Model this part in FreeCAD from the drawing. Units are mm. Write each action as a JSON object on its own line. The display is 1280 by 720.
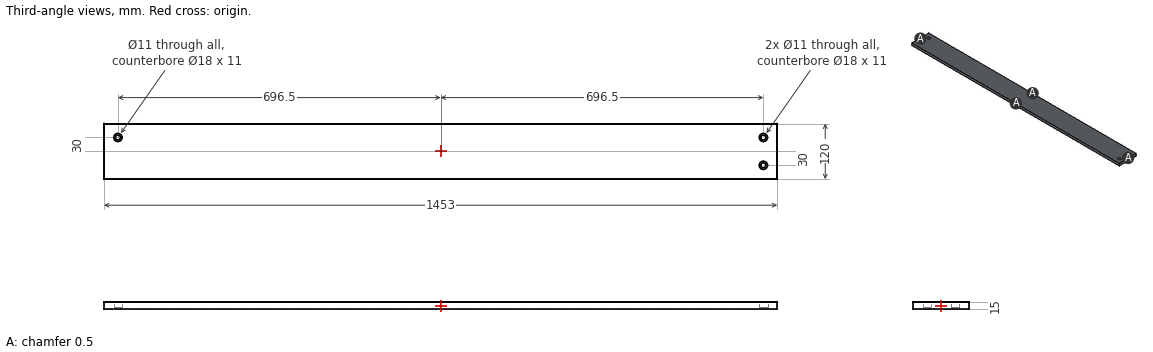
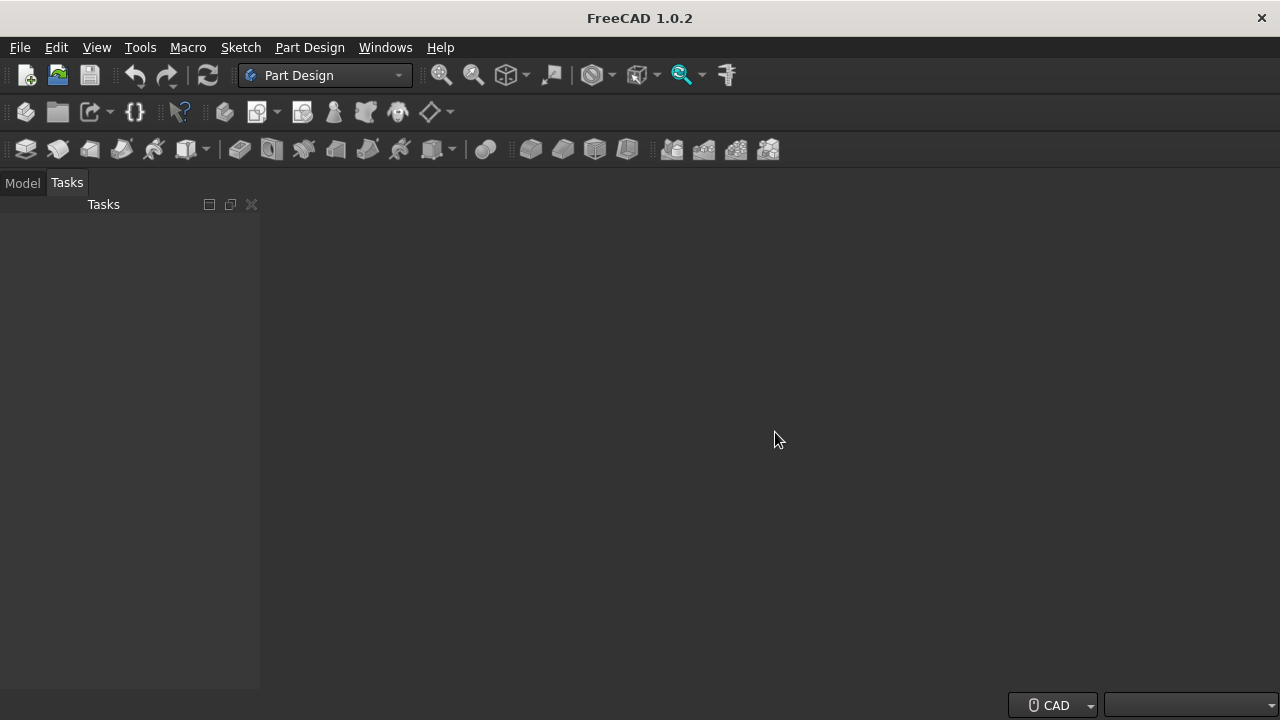
{"action": "left_click", "coordinate": [26, 76]}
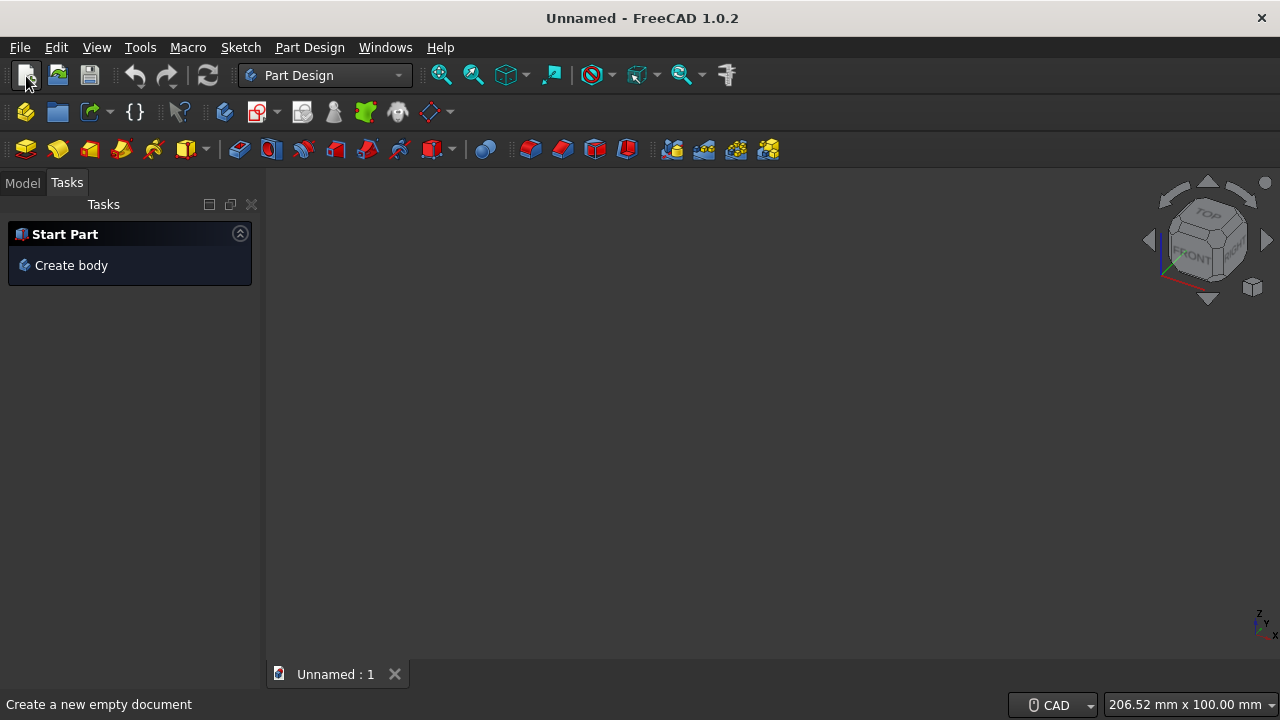
{"action": "left_click", "coordinate": [258, 112]}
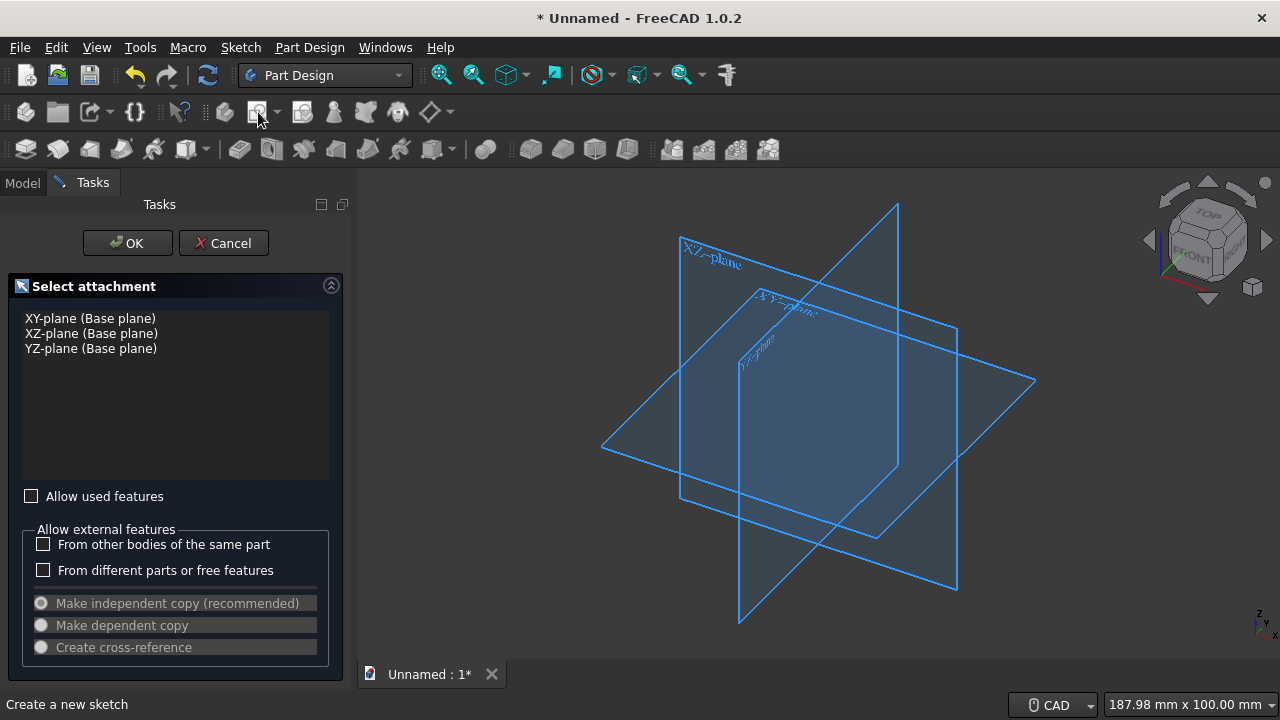
{"action": "left_click", "coordinate": [82, 318]}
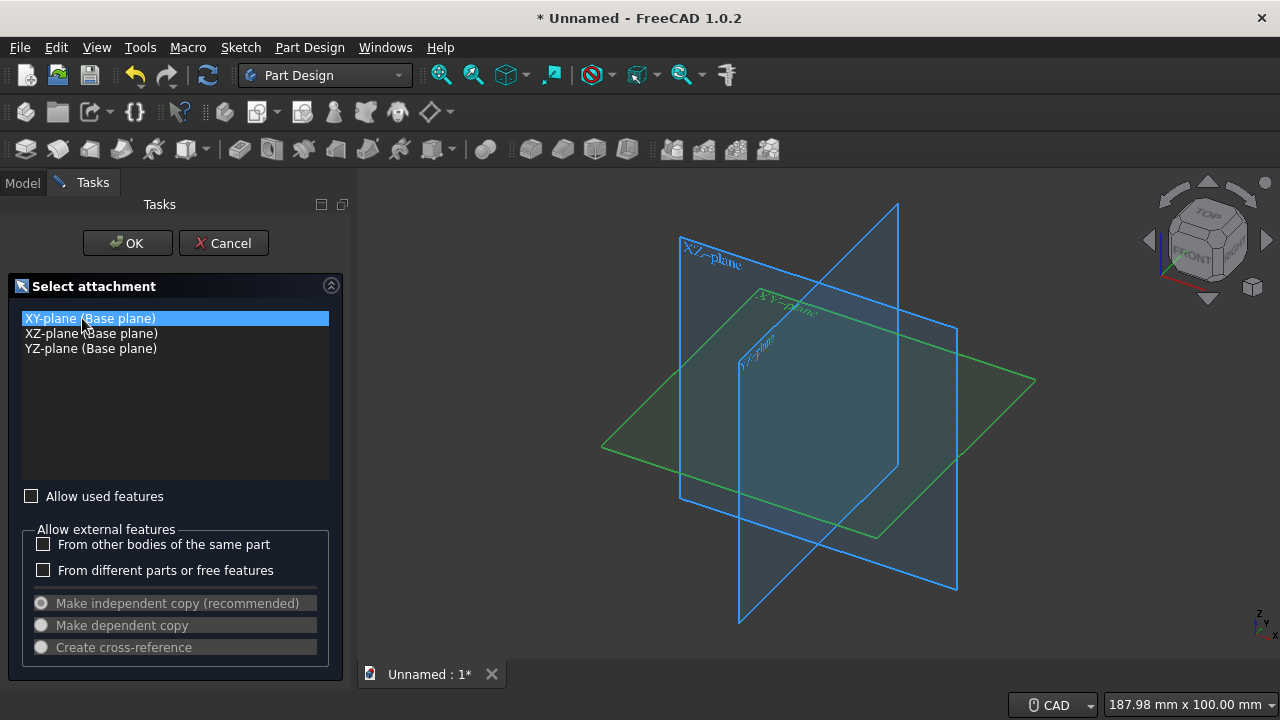
{"action": "left_click", "coordinate": [128, 243]}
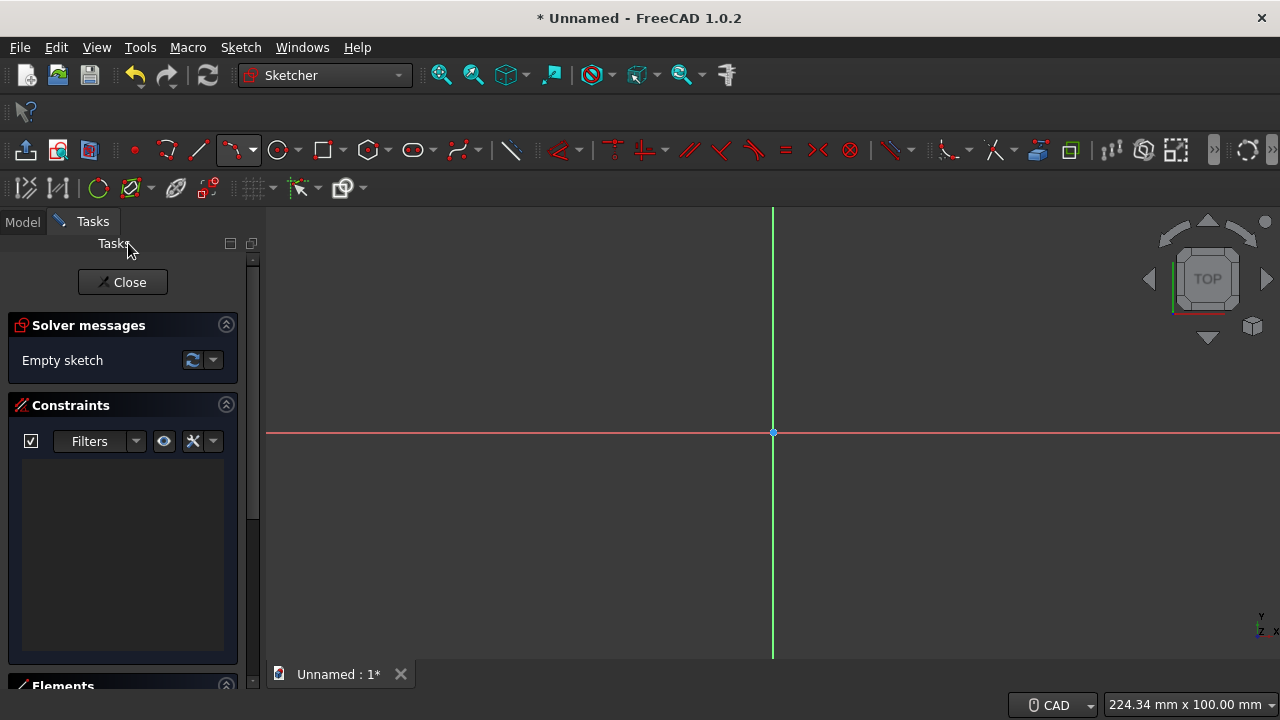
{"action": "scroll", "coordinate": [698, 433], "scroll_direction": "down", "scroll_amount": 12}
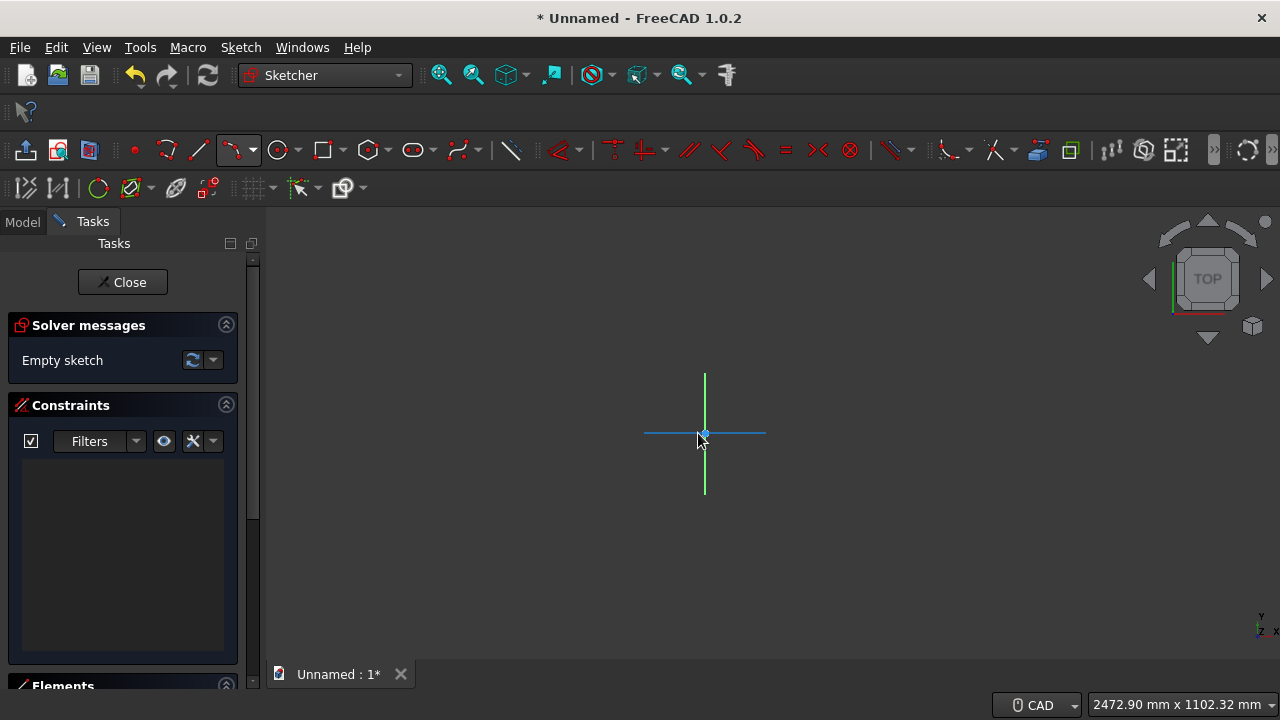
{"action": "left_click", "coordinate": [346, 150]}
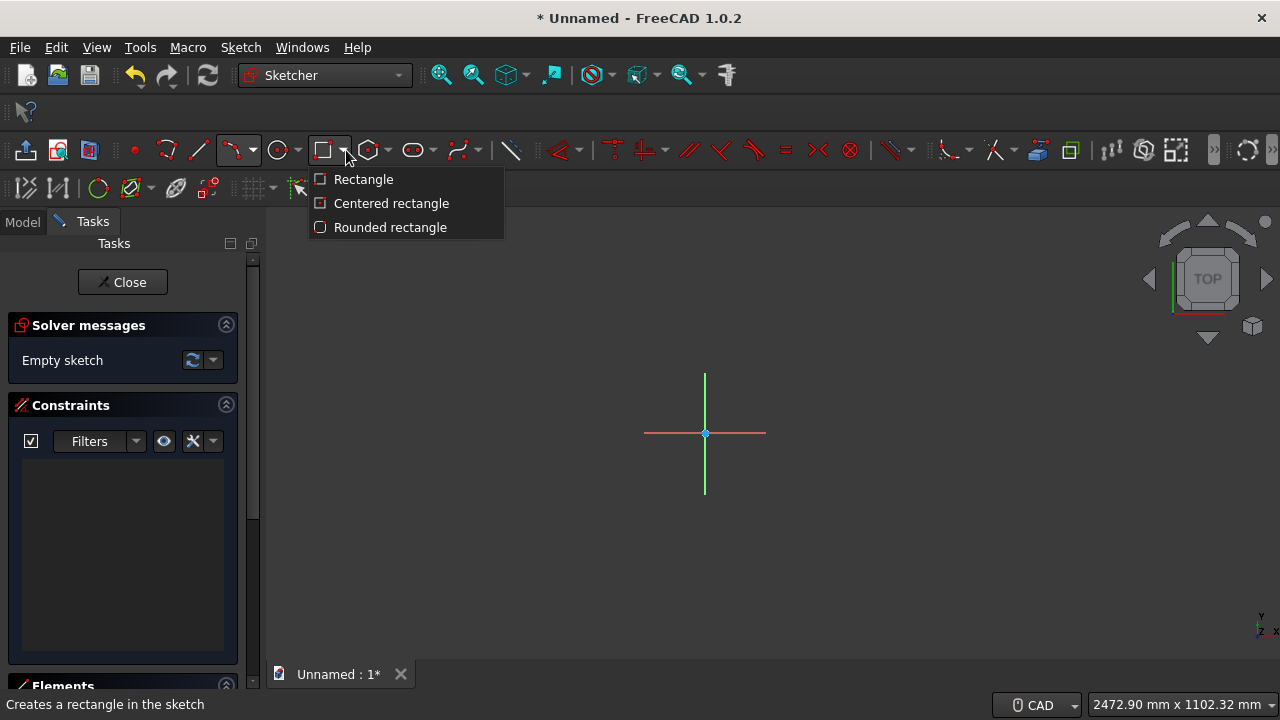
{"action": "left_click", "coordinate": [406, 203]}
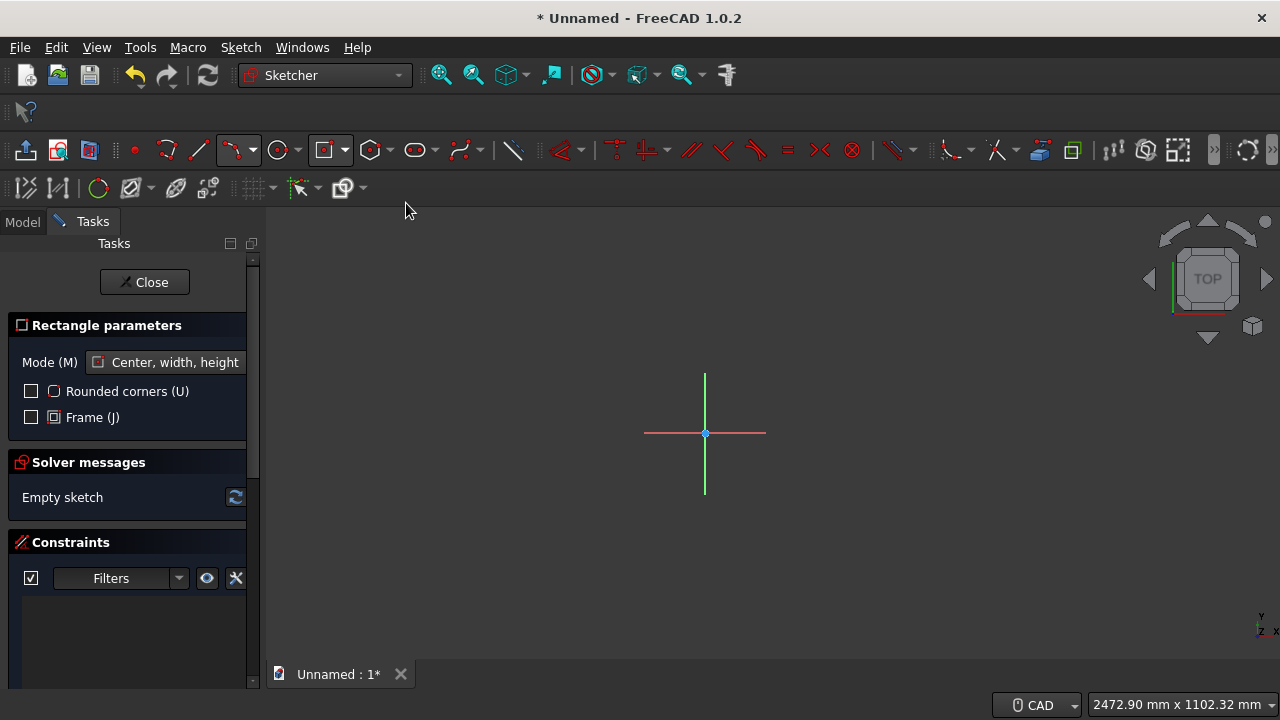
{"action": "left_click", "coordinate": [705, 433]}
{"action": "mouse_move", "coordinate": [1003, 409]}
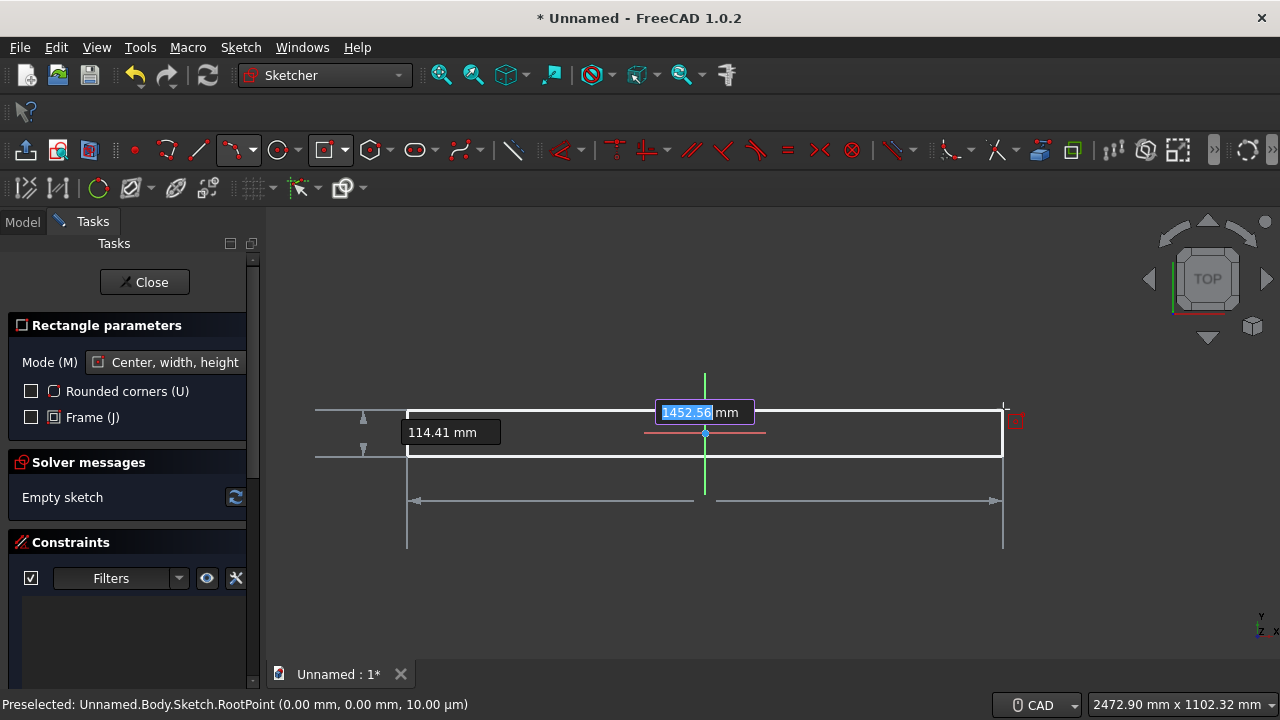
{"action": "type", "text": "1453"}
{"action": "key", "text": "Tab"}
{"action": "type", "text": "120"}
{"action": "key", "text": "Return"}
{"action": "key", "text": "Escape"}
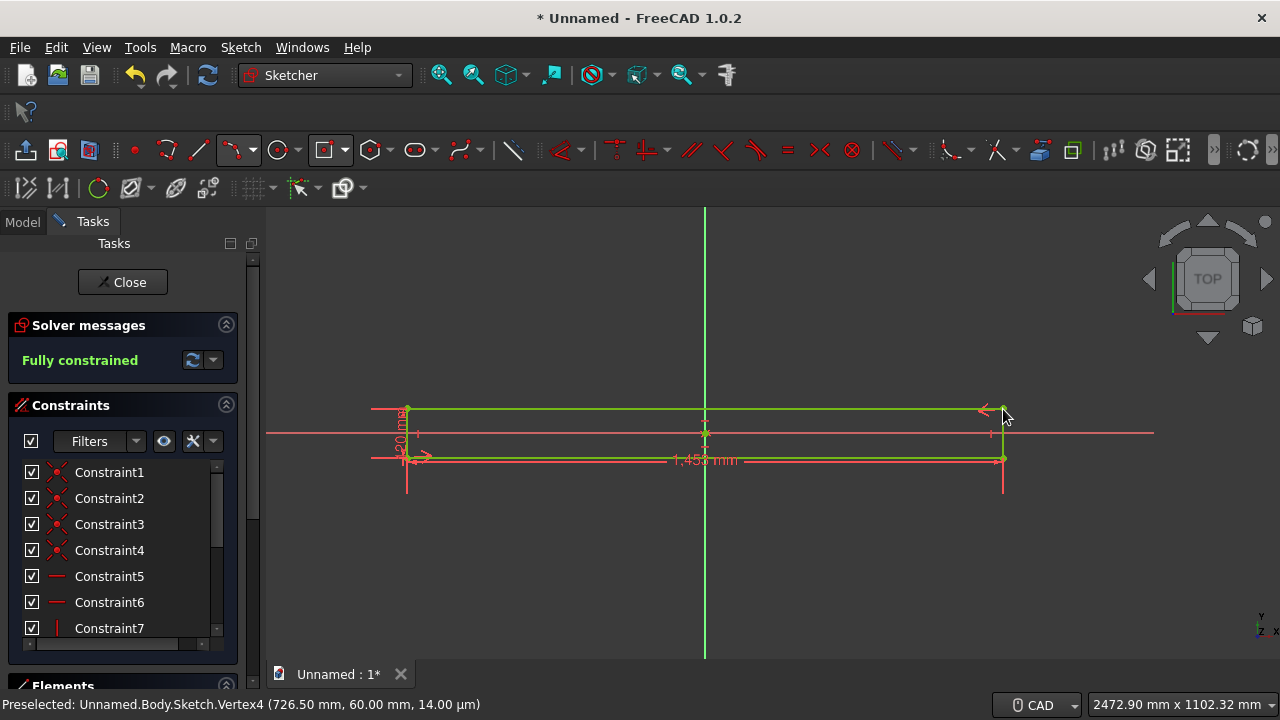
{"action": "left_click", "coordinate": [123, 282]}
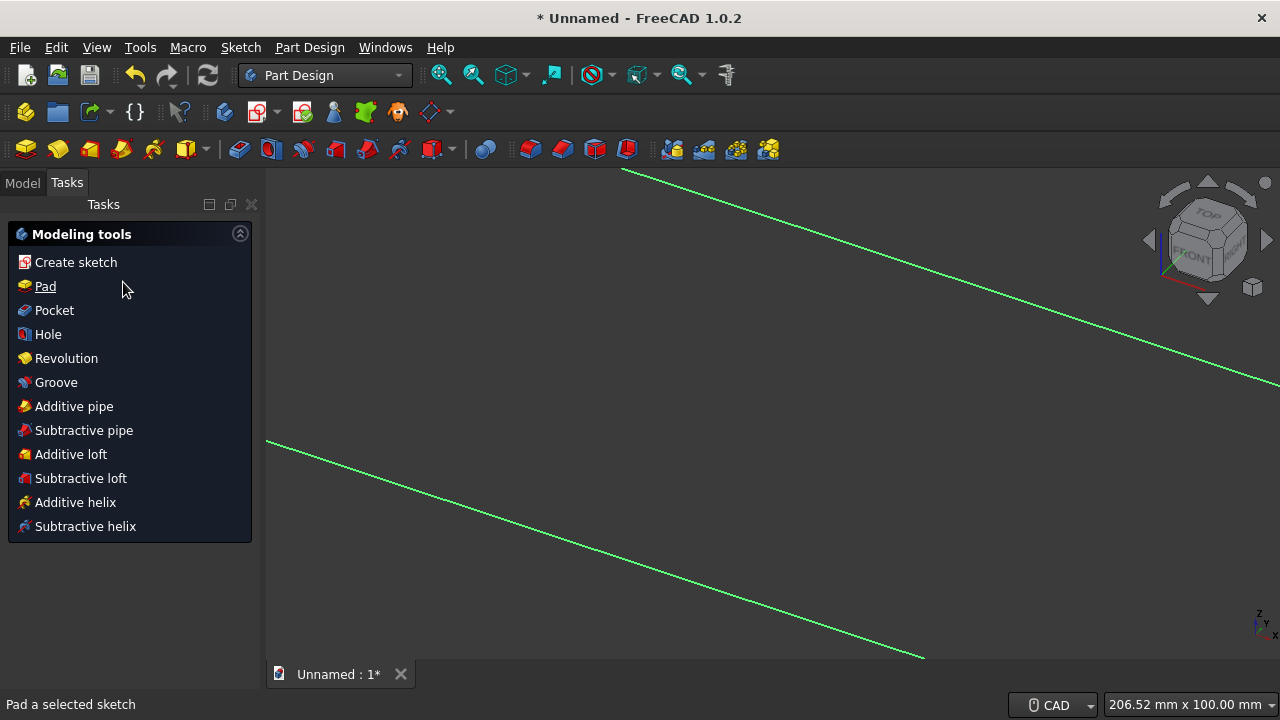
{"action": "left_click", "coordinate": [26, 150]}